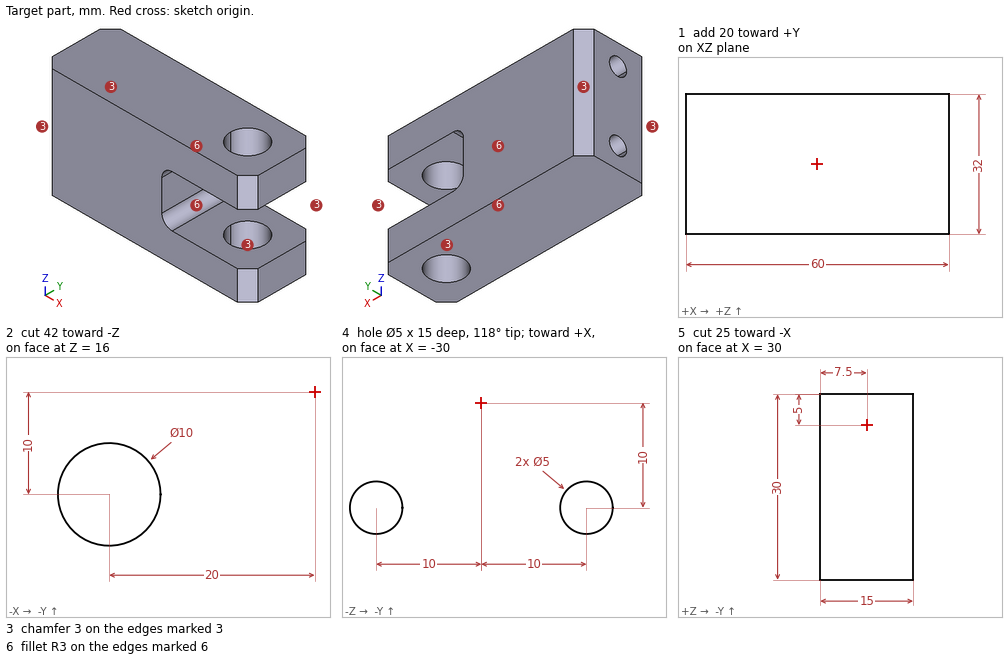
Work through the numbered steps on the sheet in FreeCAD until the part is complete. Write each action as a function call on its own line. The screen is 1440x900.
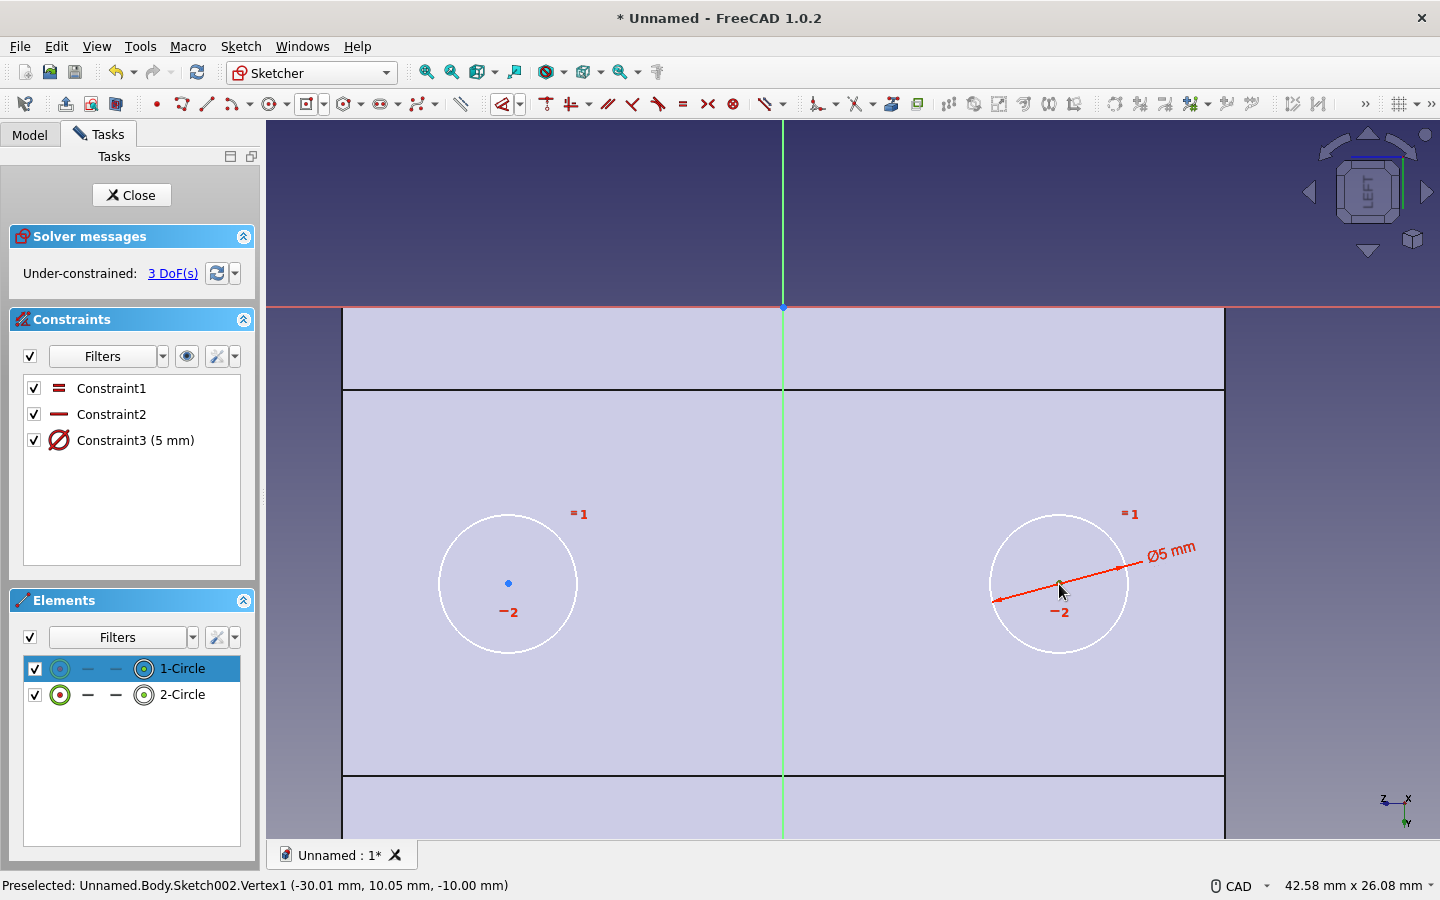
key(l)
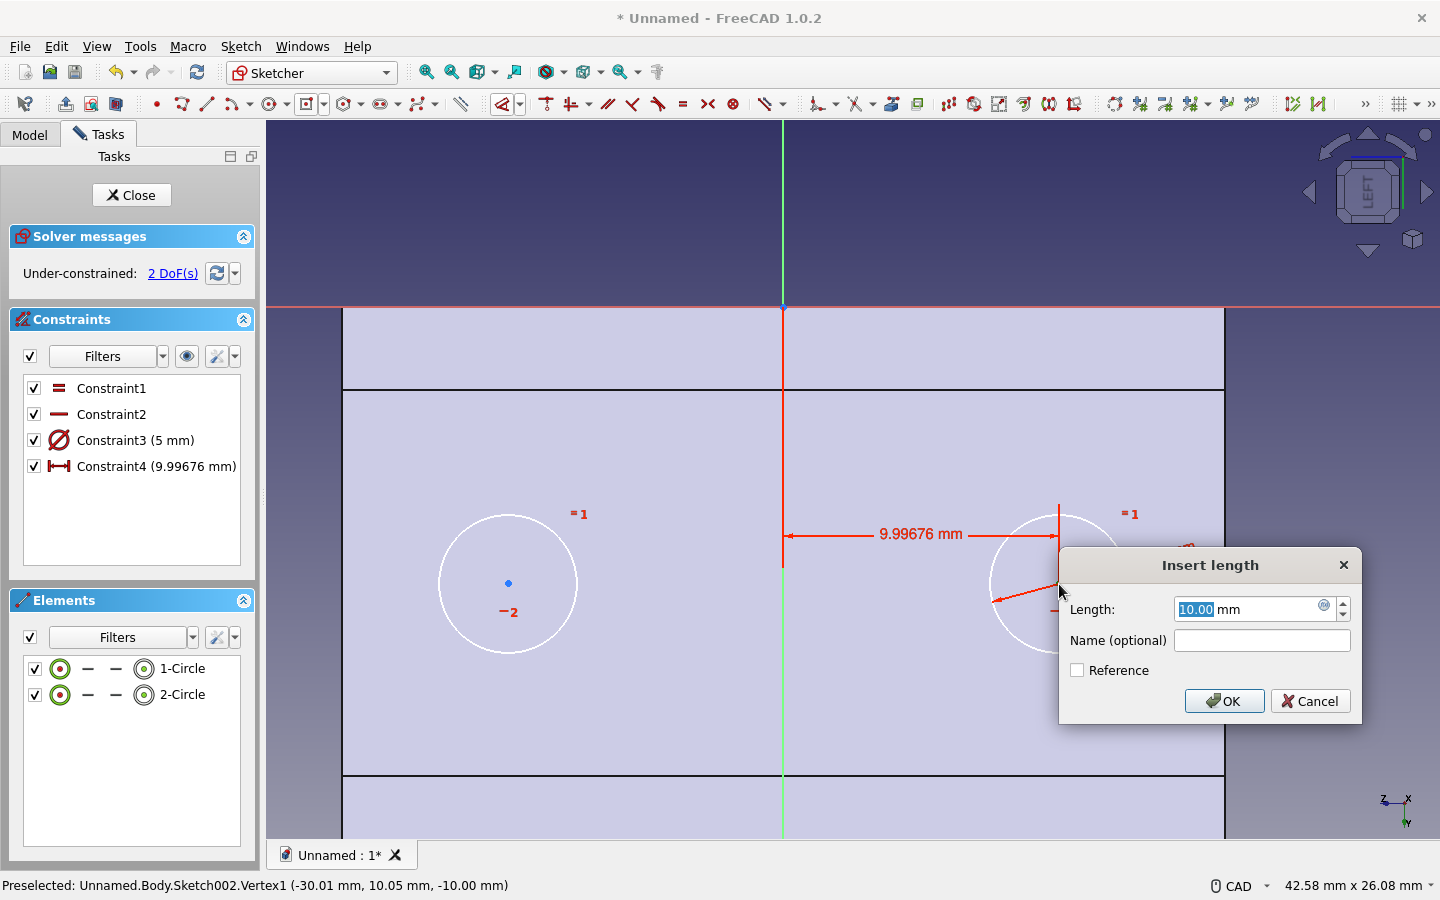
text(10)
key(Return)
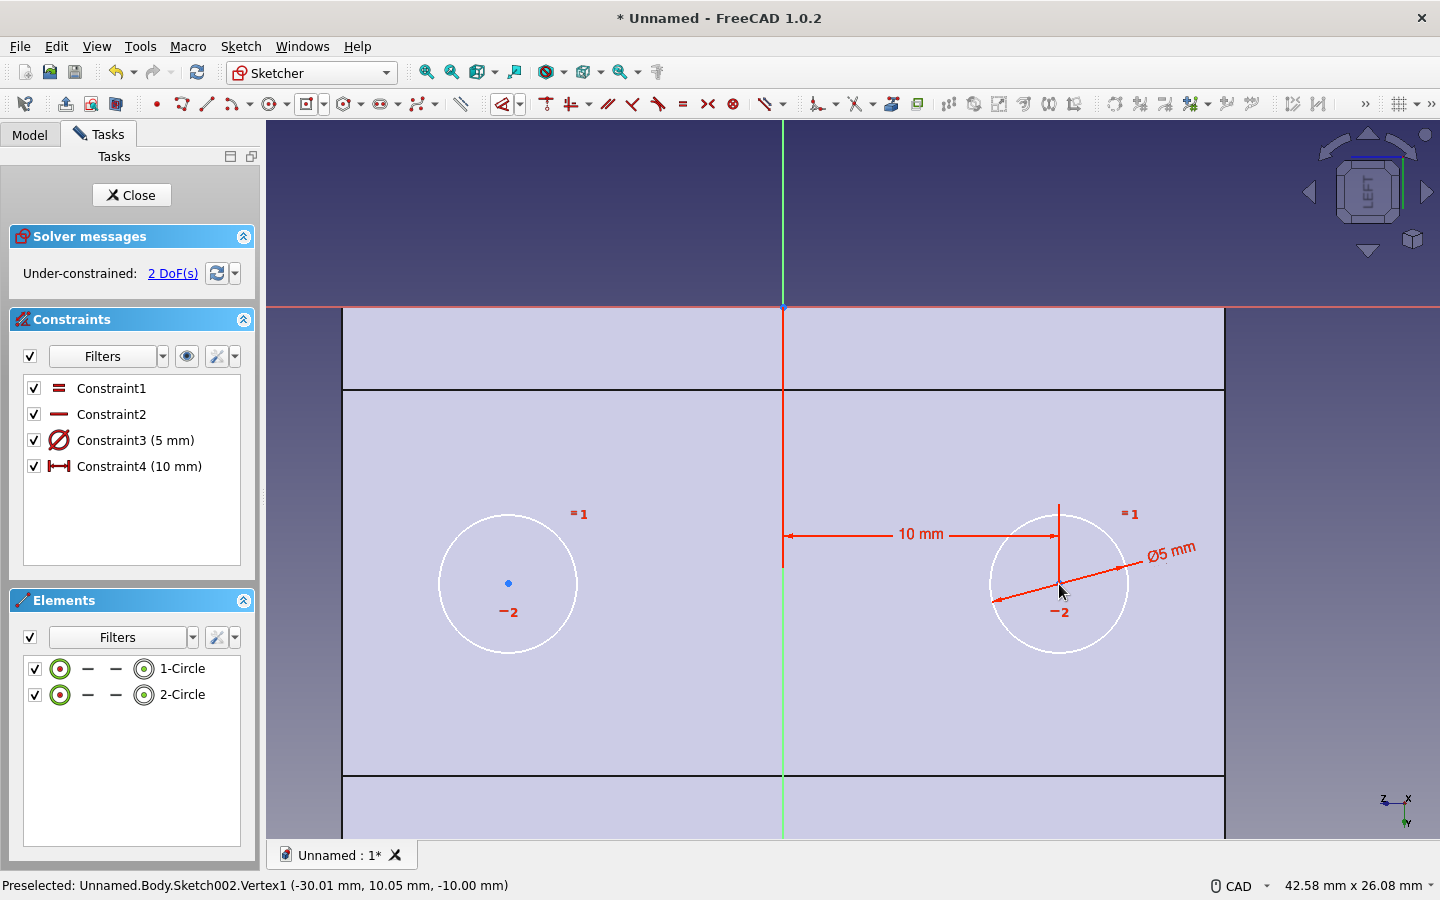
click(1059, 584)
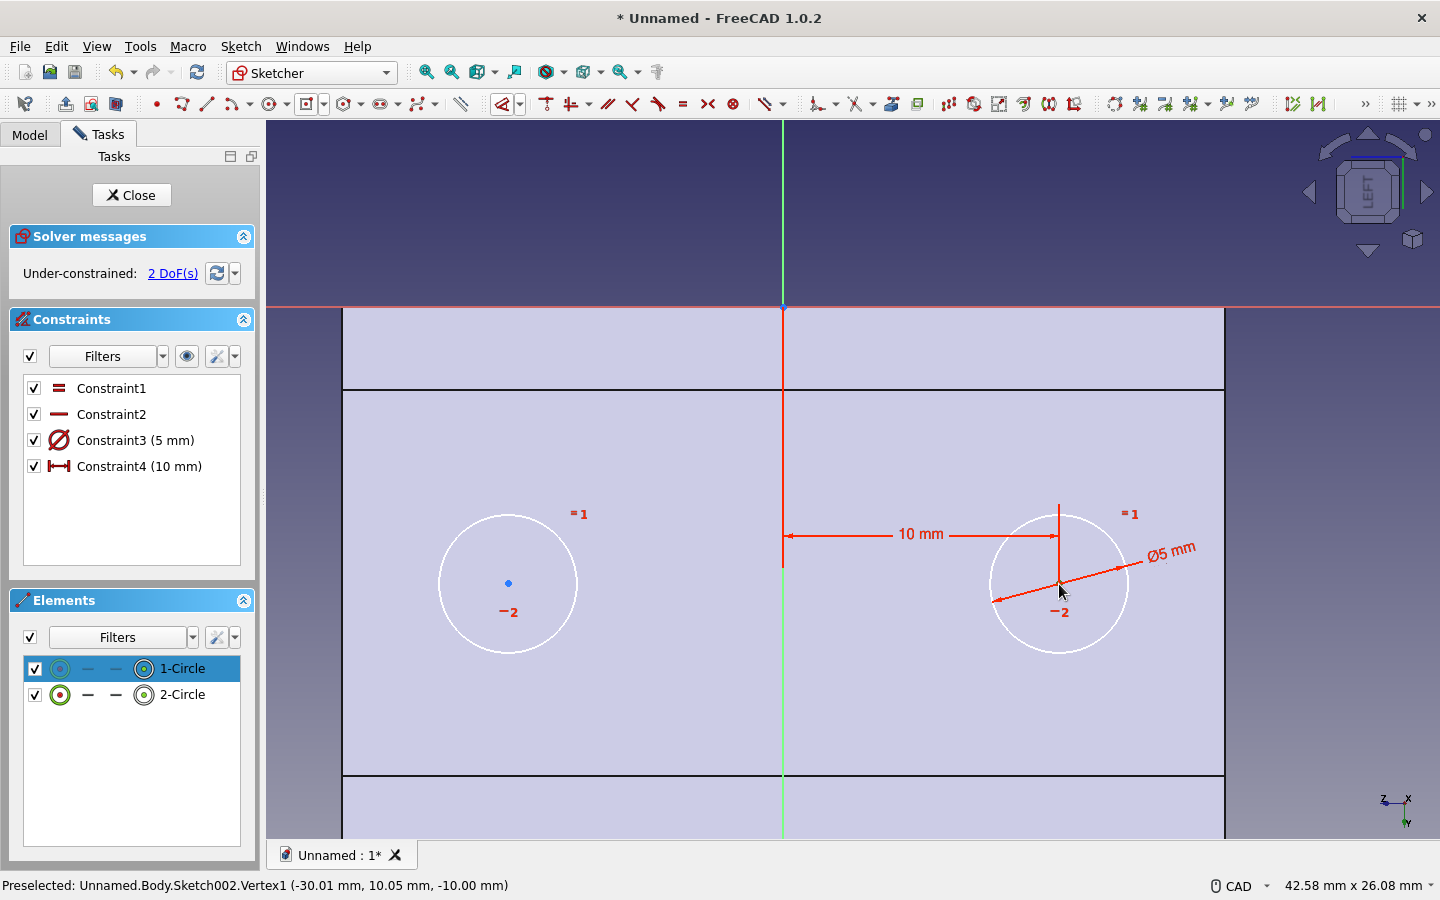
click(520, 104)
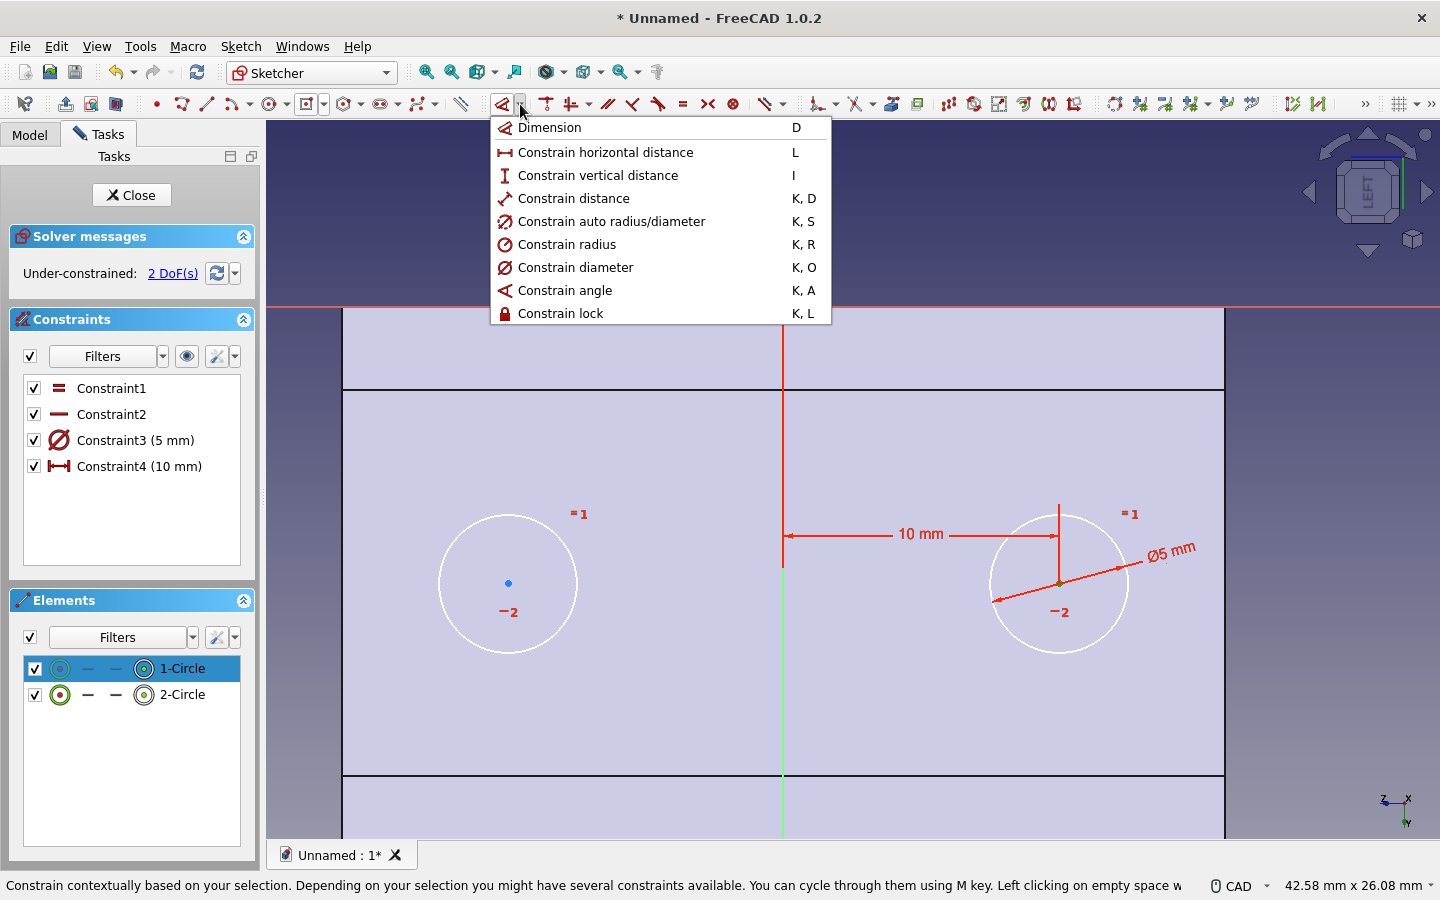
click(661, 176)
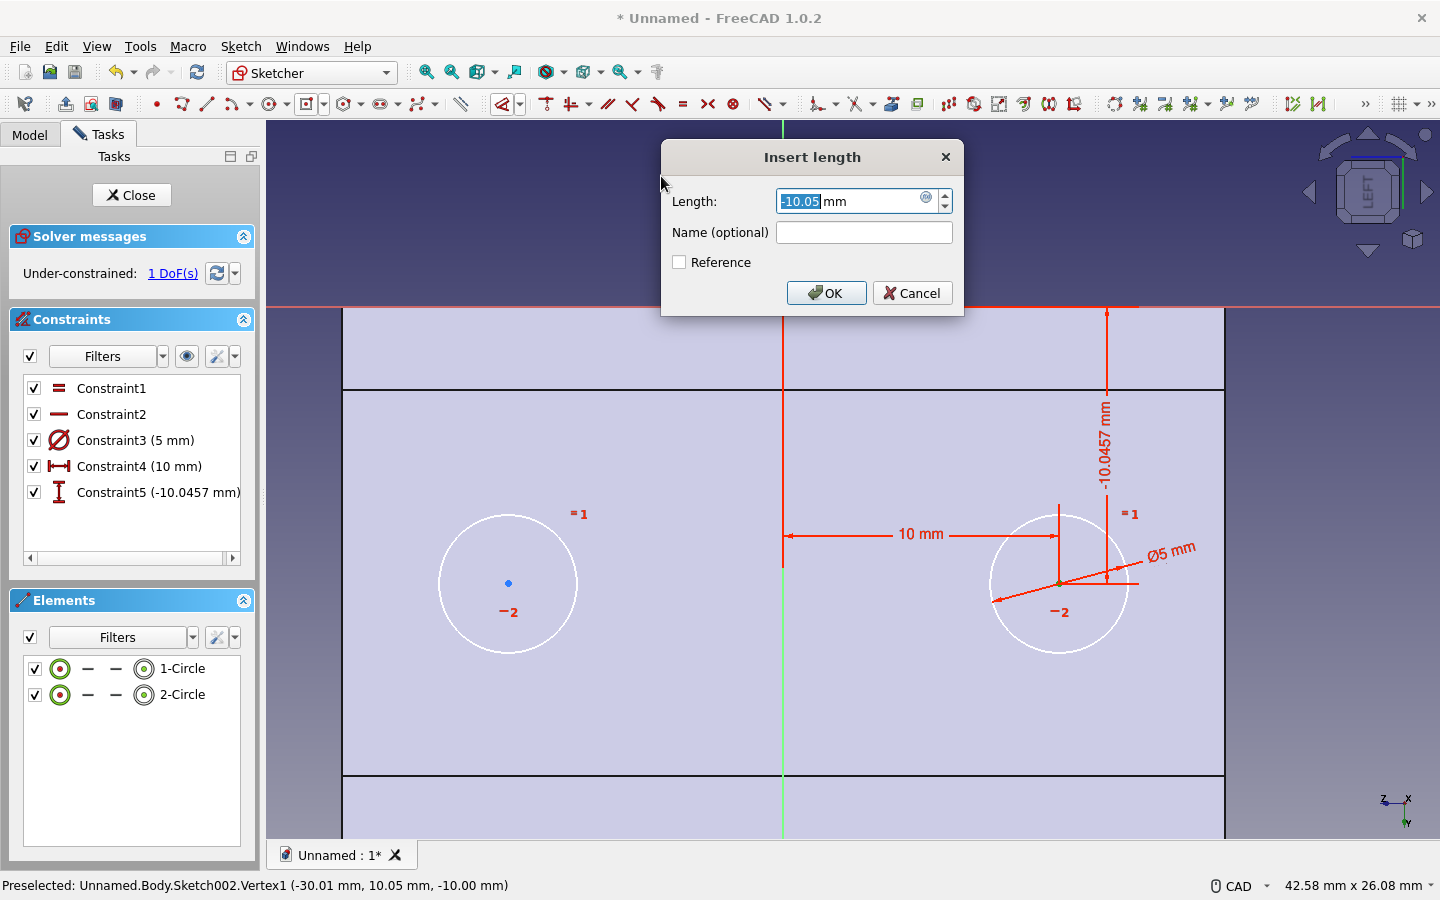
text(-10)
key(Return)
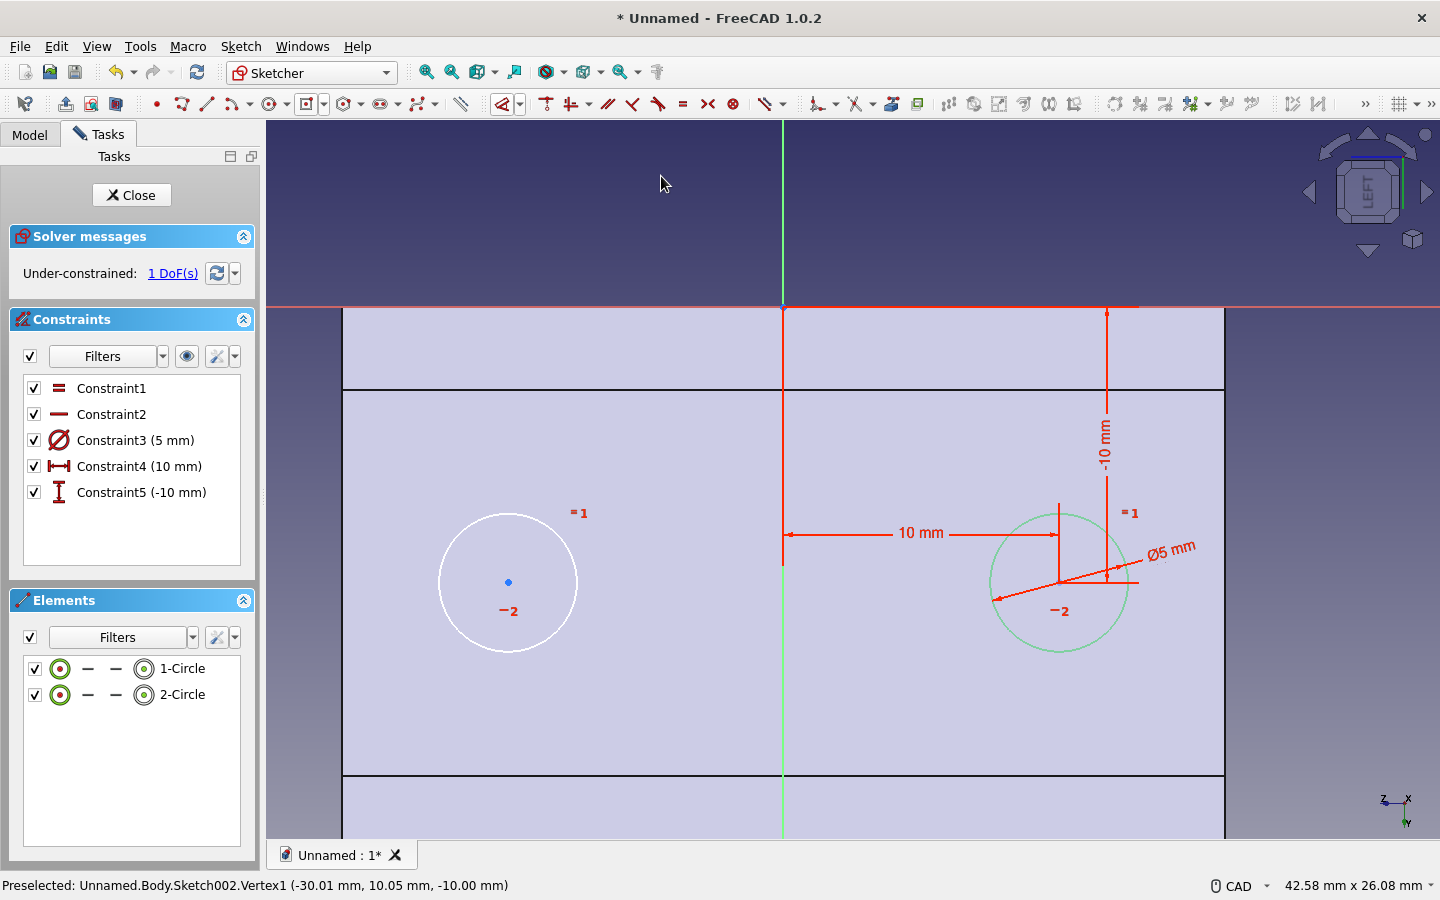
click(508, 583)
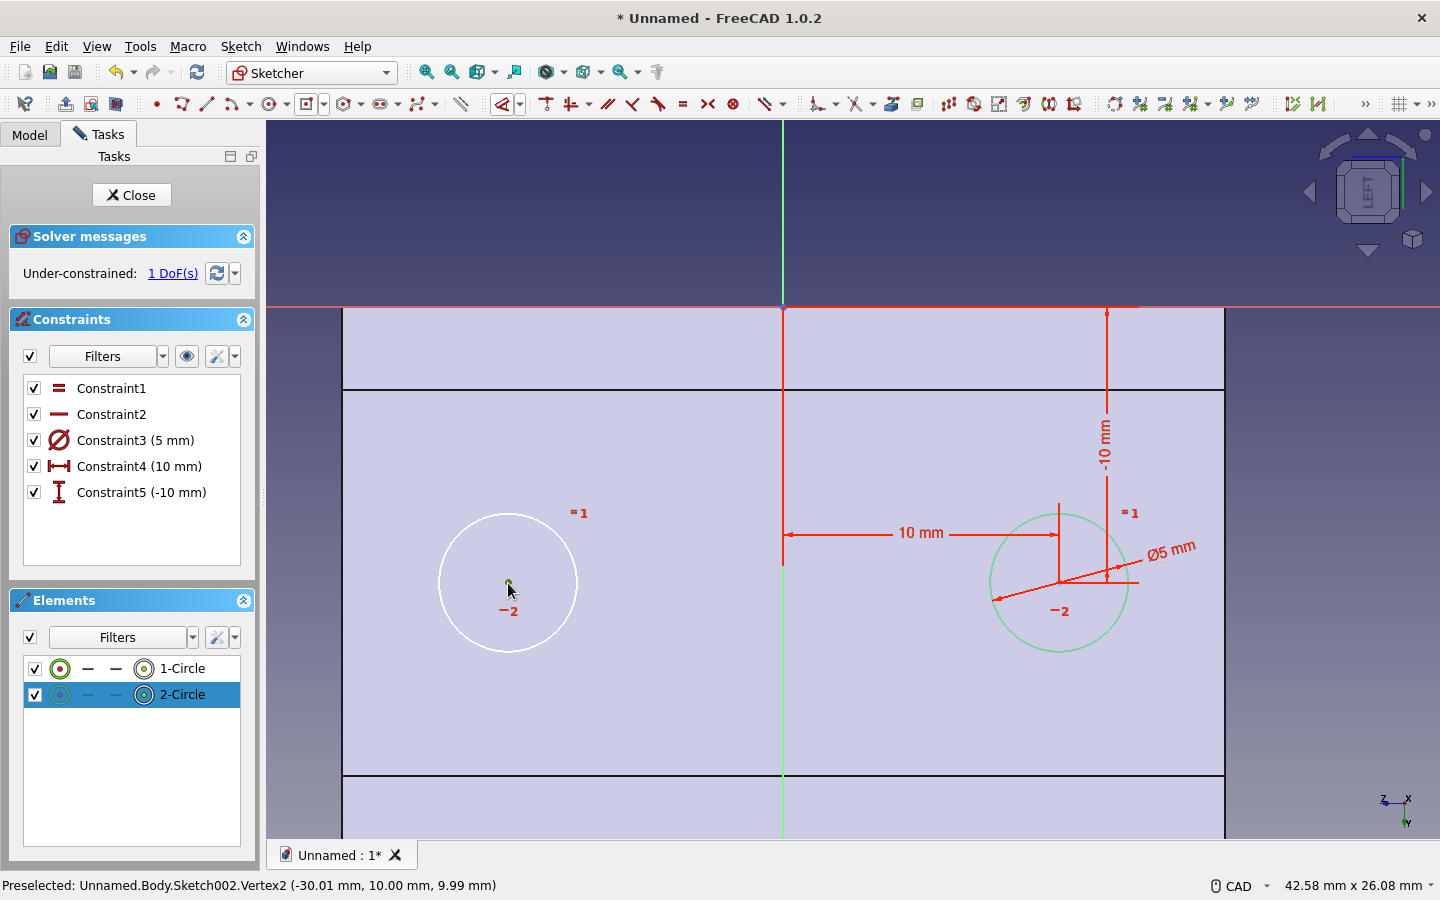
click(520, 104)